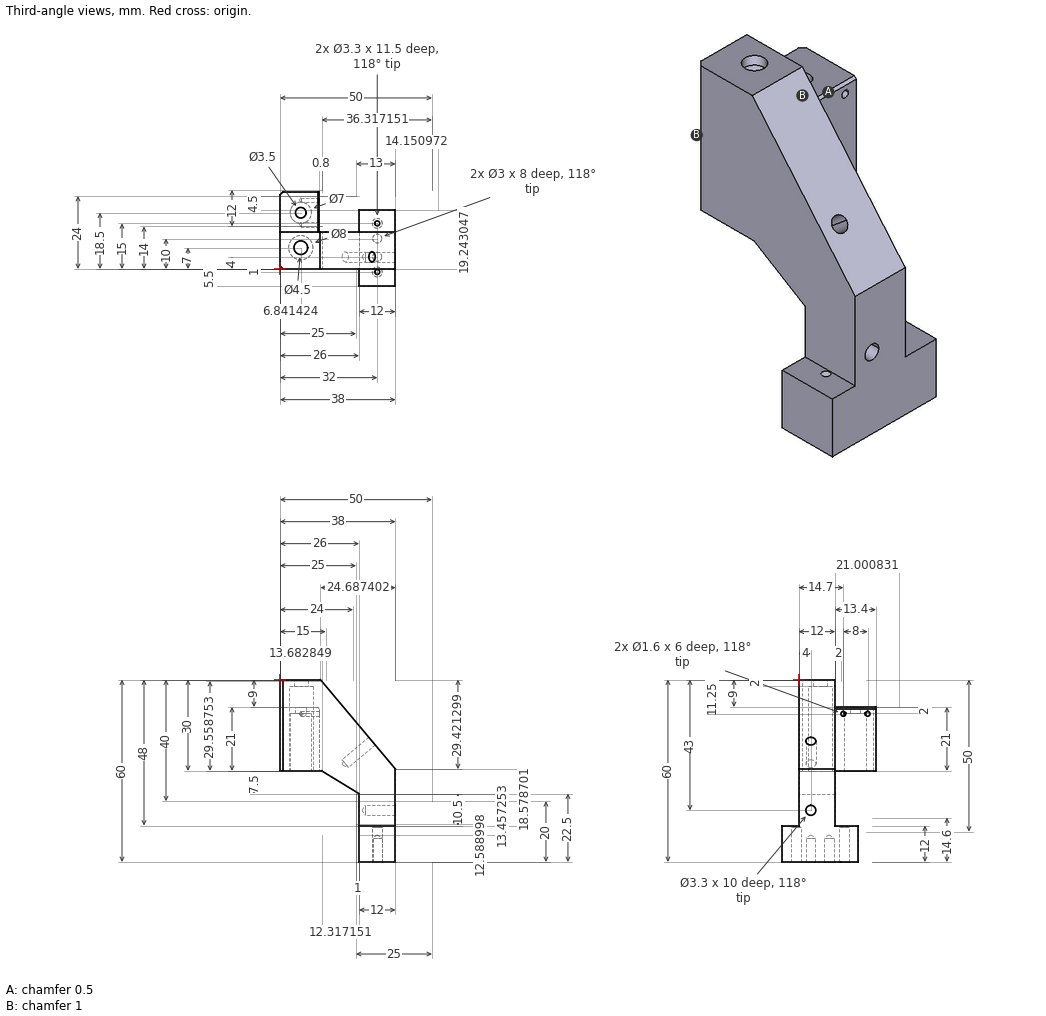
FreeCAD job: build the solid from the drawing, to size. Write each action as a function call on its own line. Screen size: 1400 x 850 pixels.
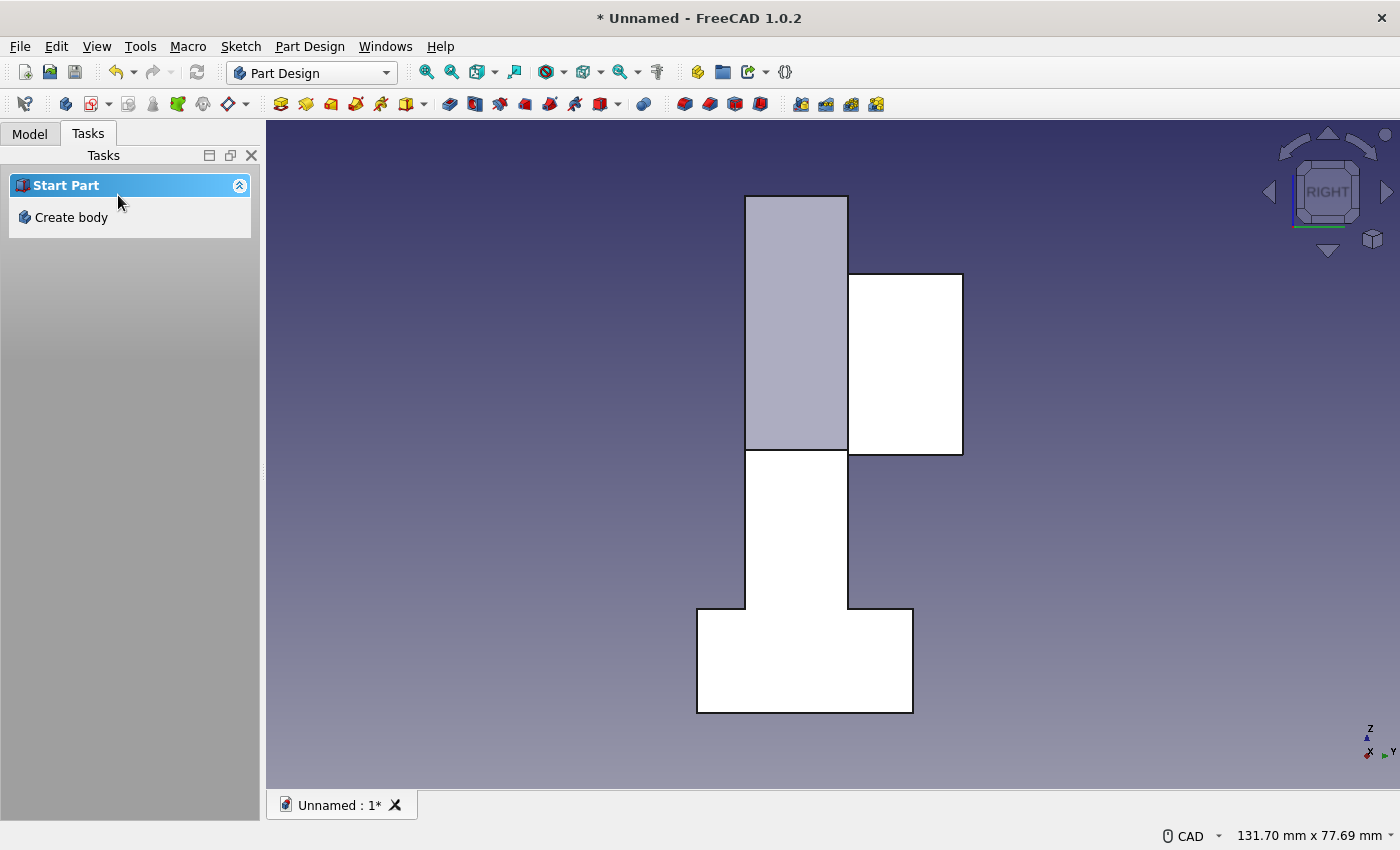
key(5)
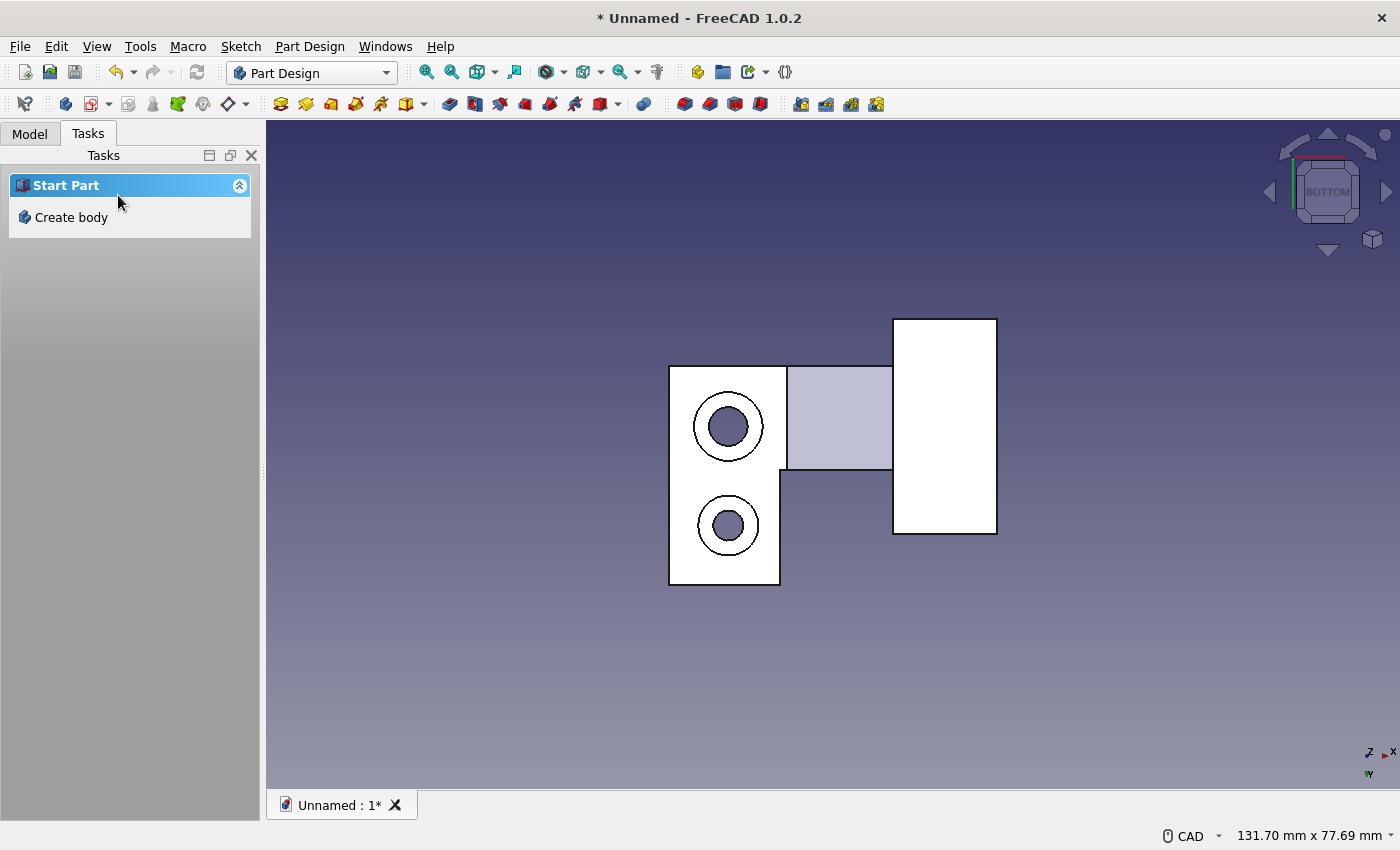
click(427, 72)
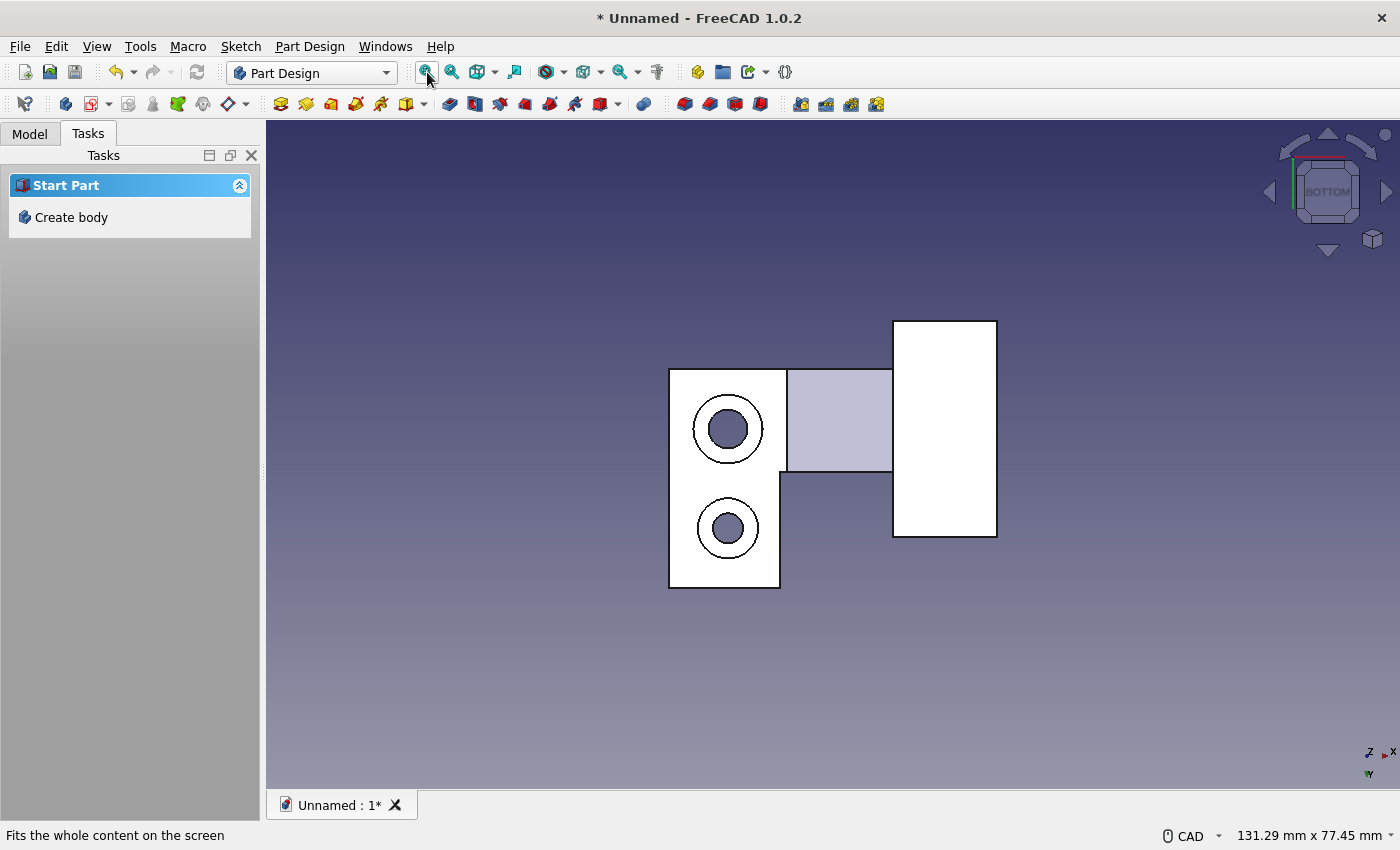
click(945, 459)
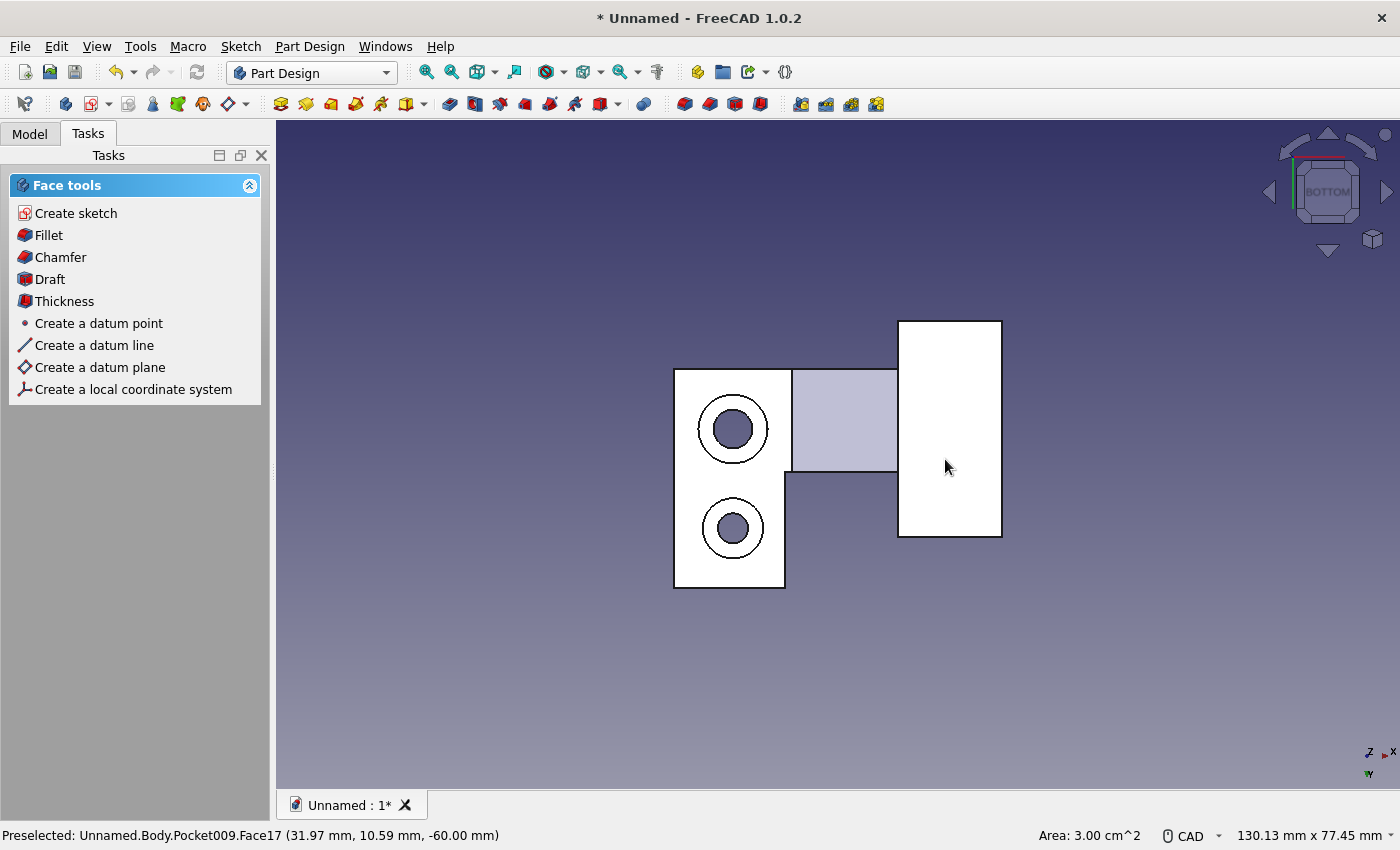
click(90, 104)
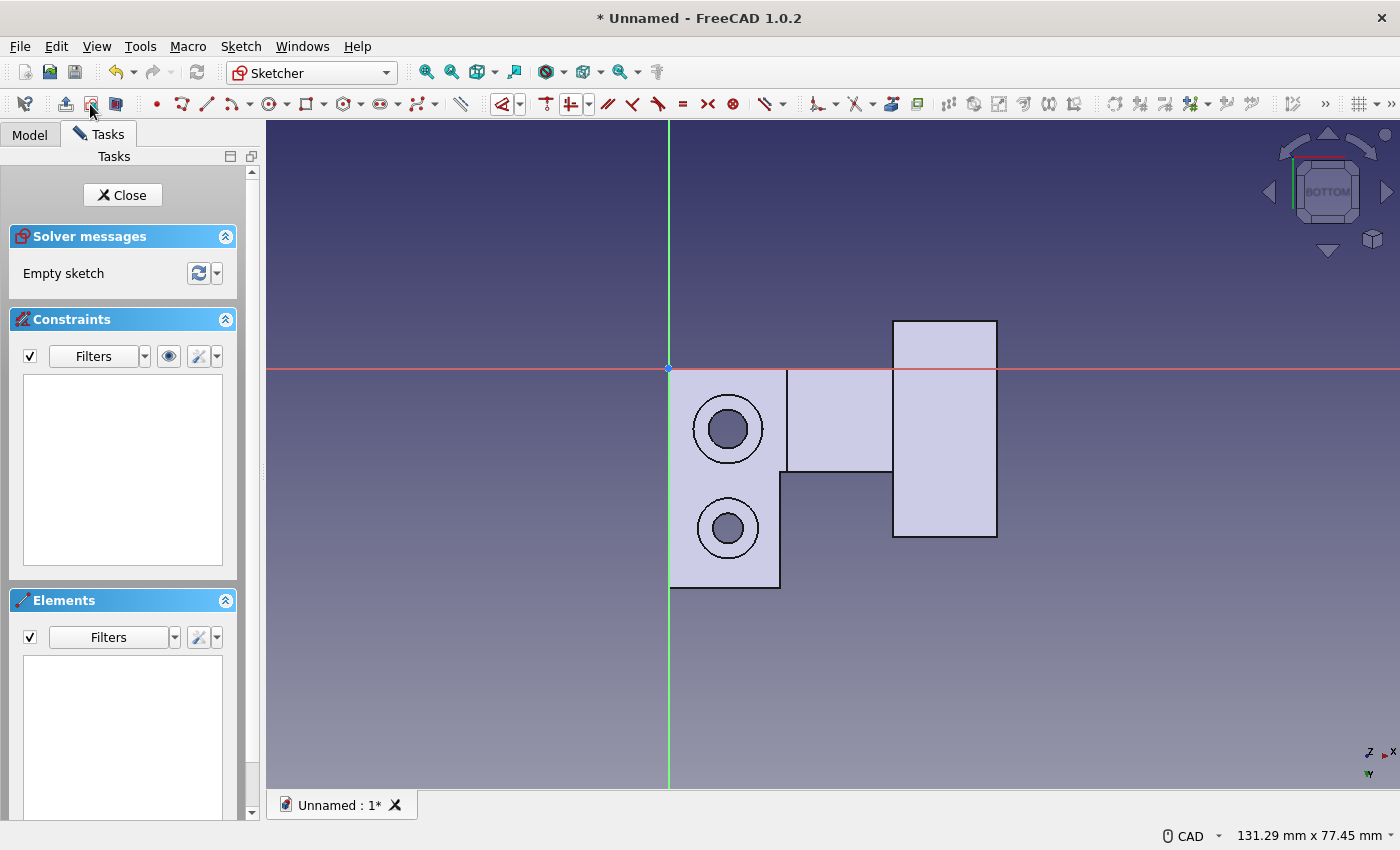
scroll(855, 408, up, 4)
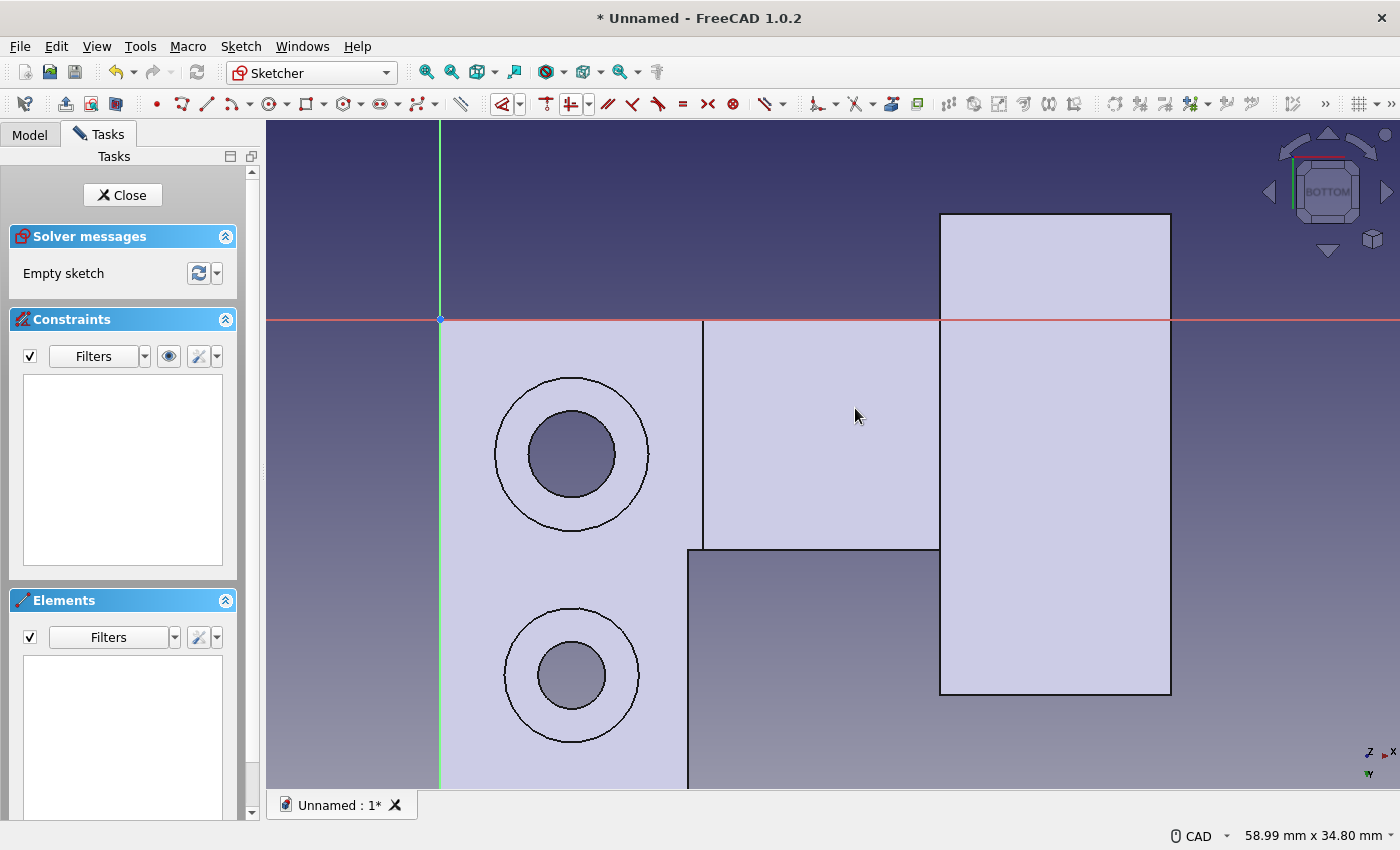
key(g)
key(c)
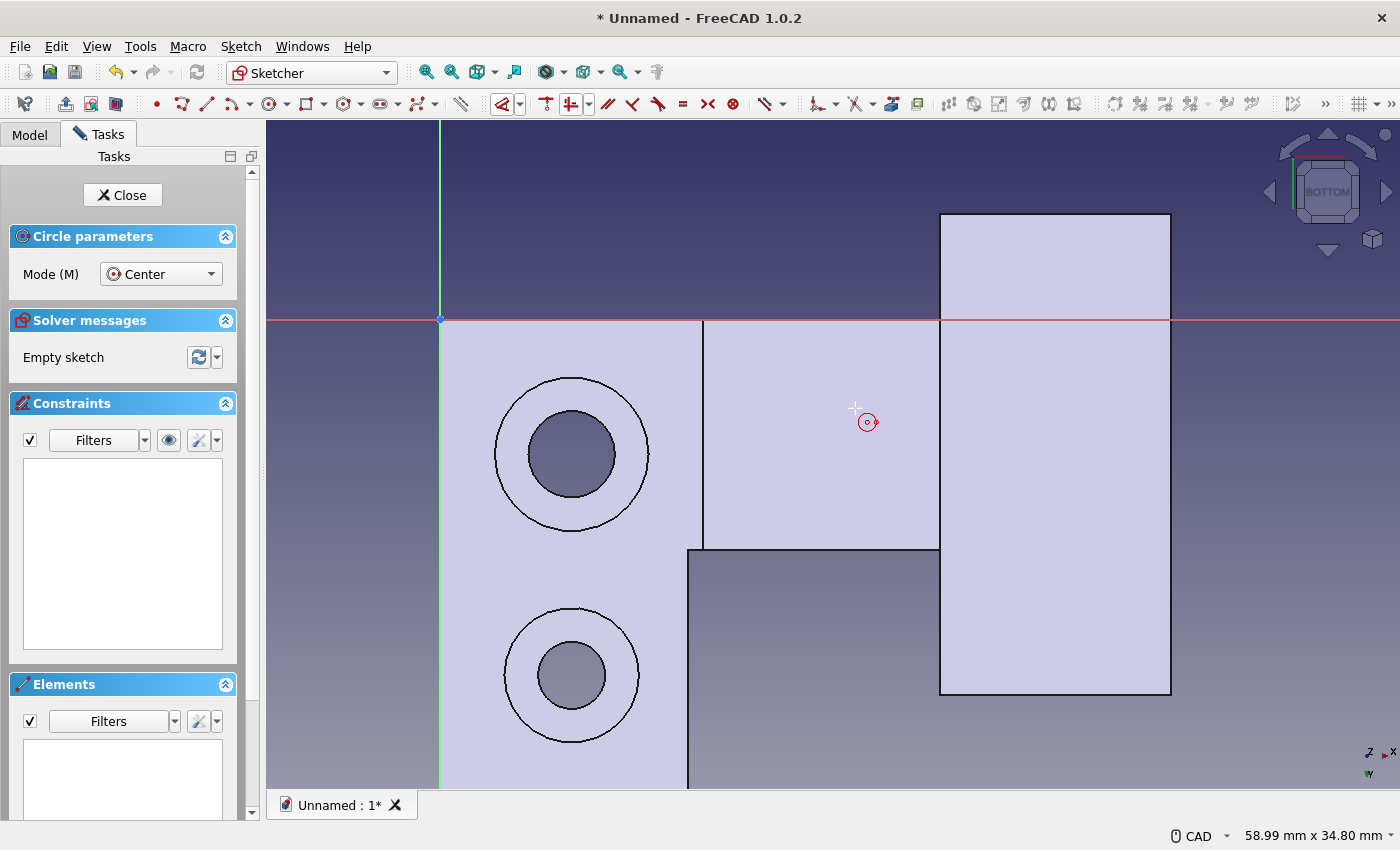
click(1055, 608)
click(1078, 586)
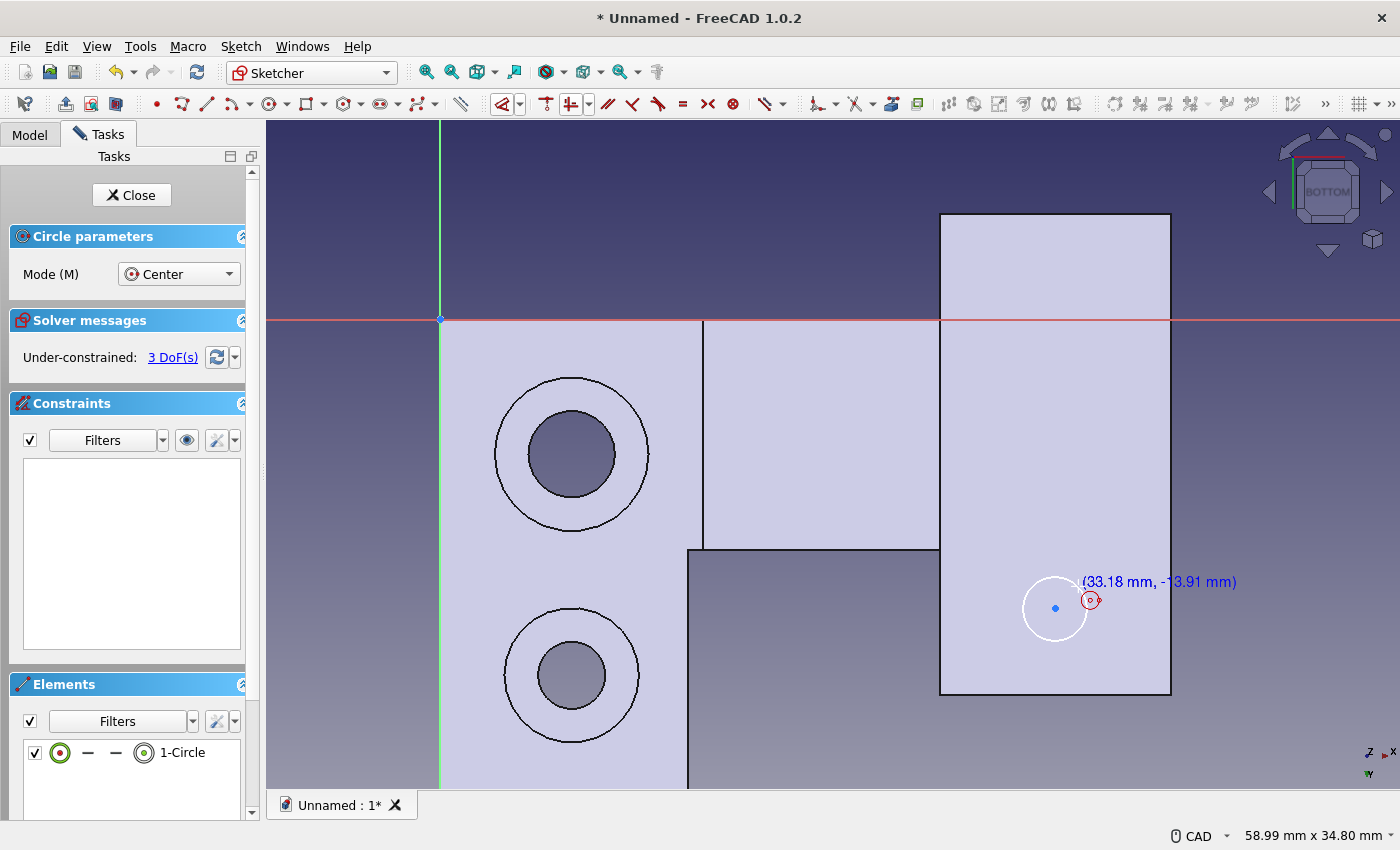
click(1055, 300)
click(1078, 278)
key(Escape)